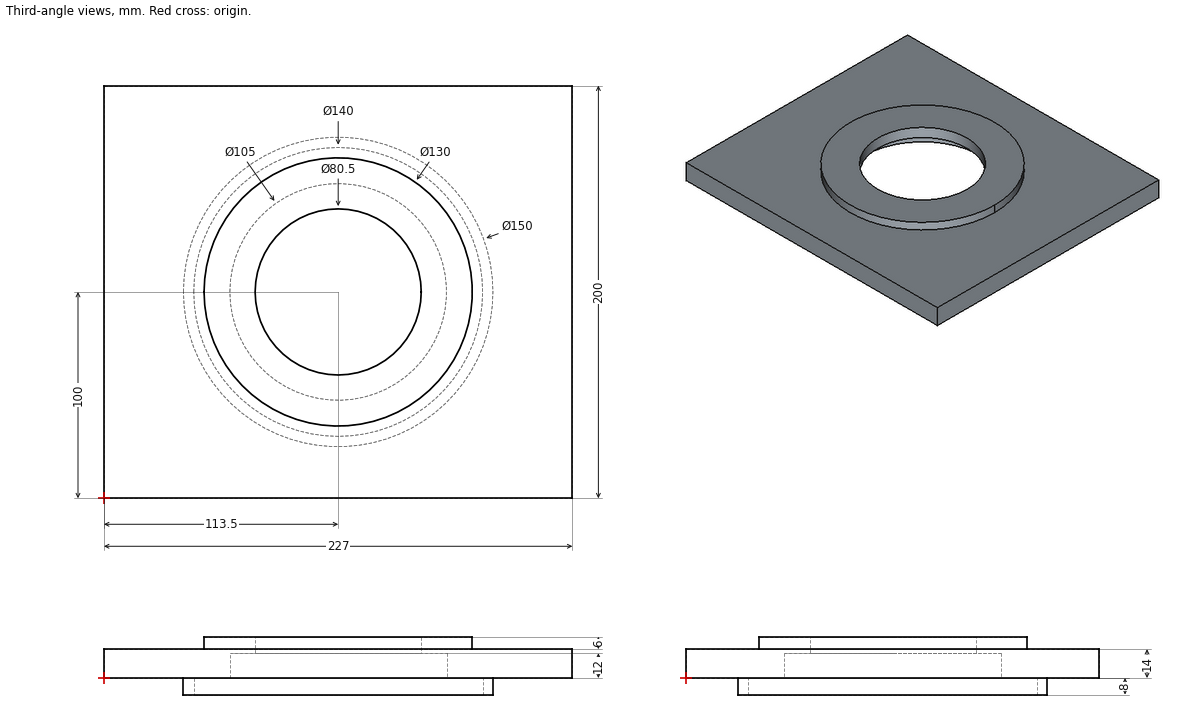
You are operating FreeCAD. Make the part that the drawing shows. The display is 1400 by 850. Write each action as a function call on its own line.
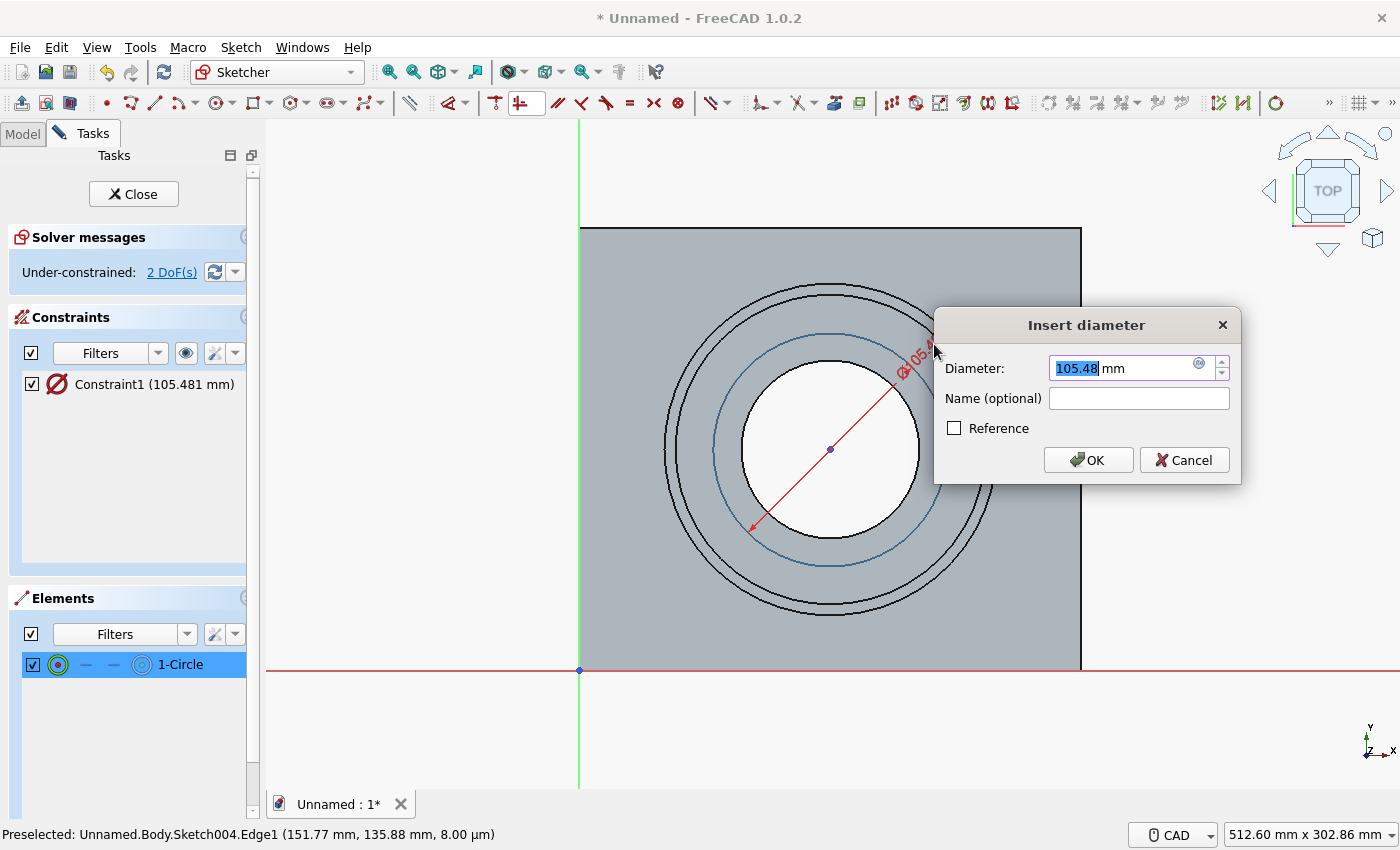
text(105)
key(Return)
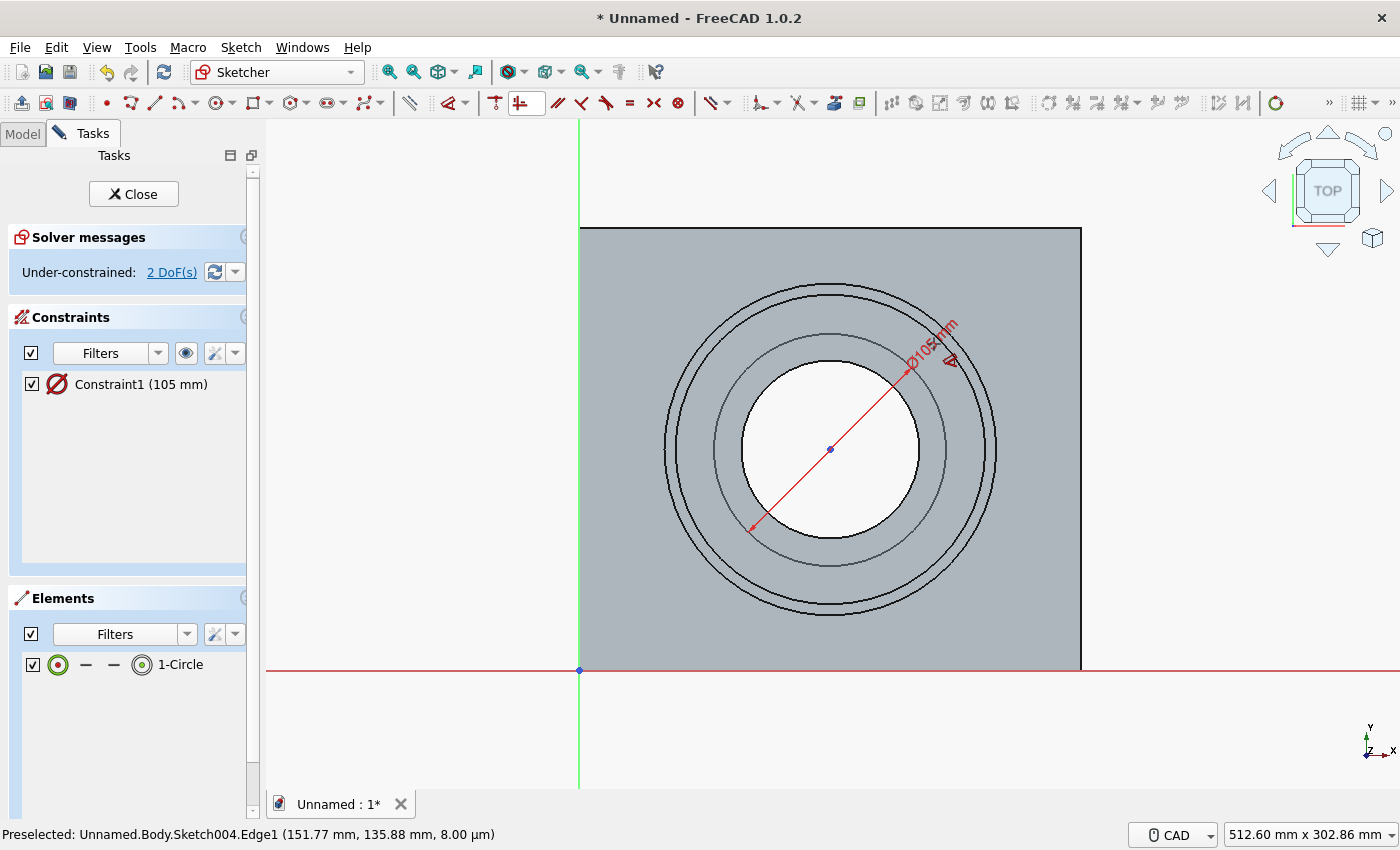
click(830, 450)
click(545, 560)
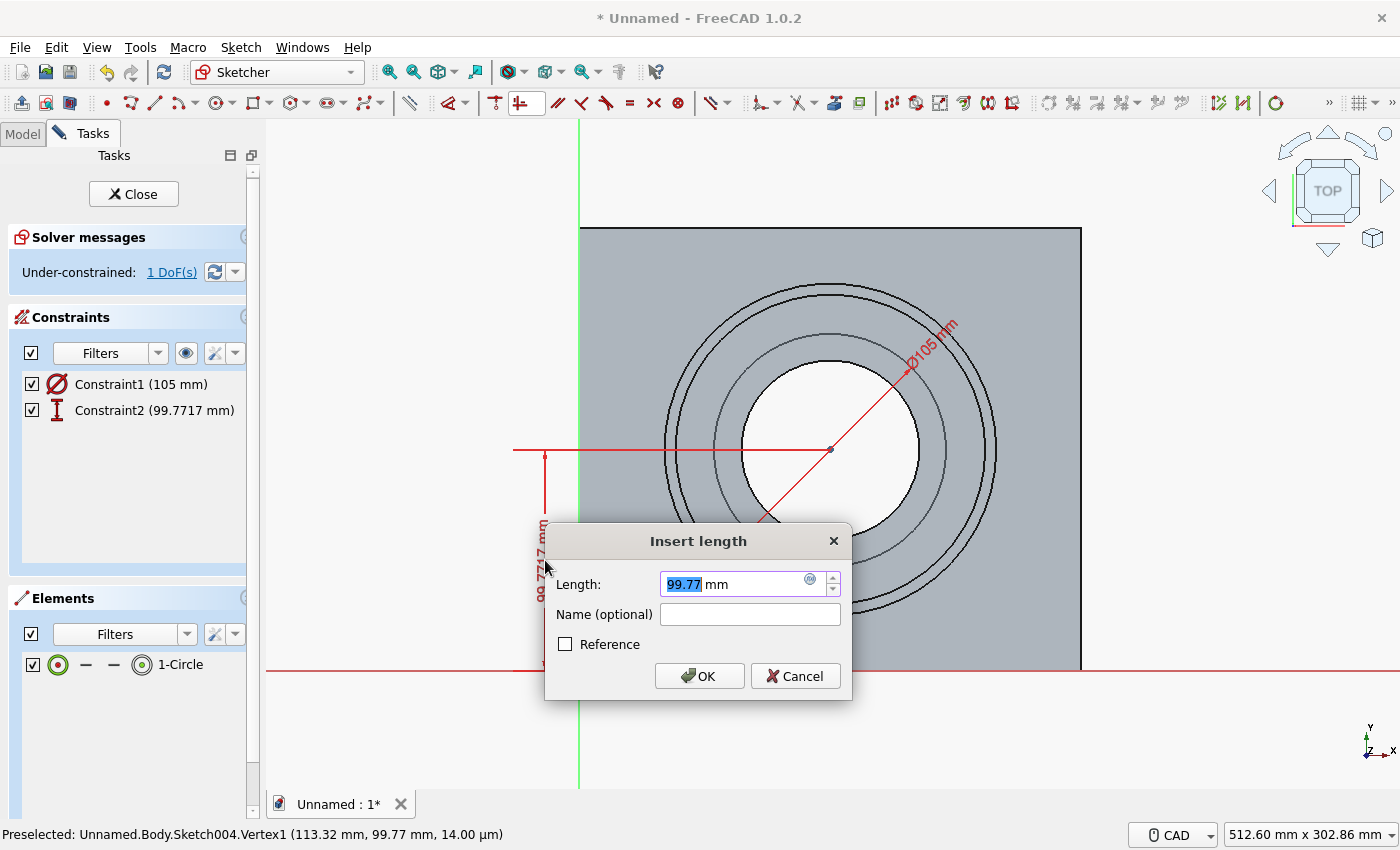
text(100)
key(Return)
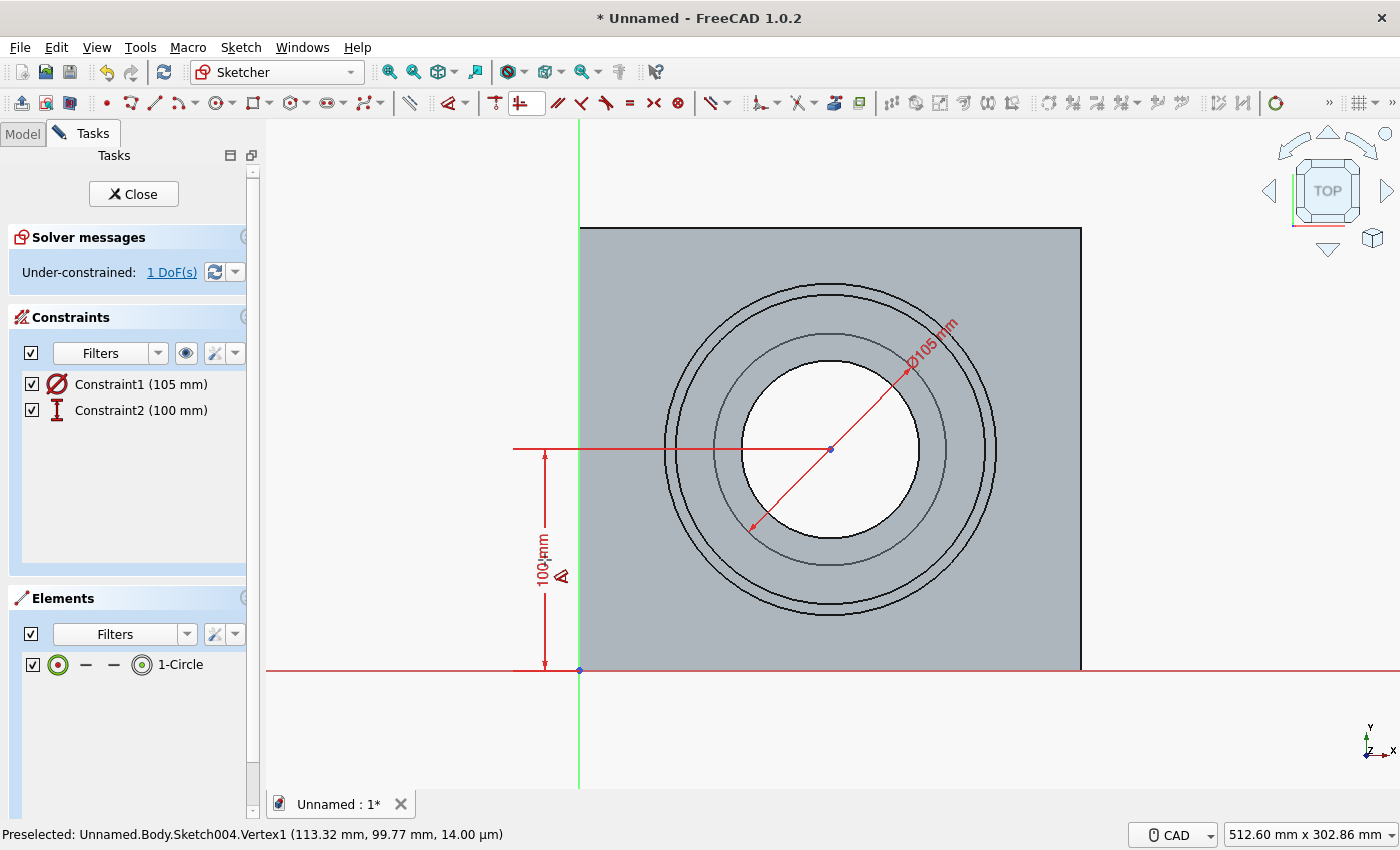
click(830, 449)
click(705, 705)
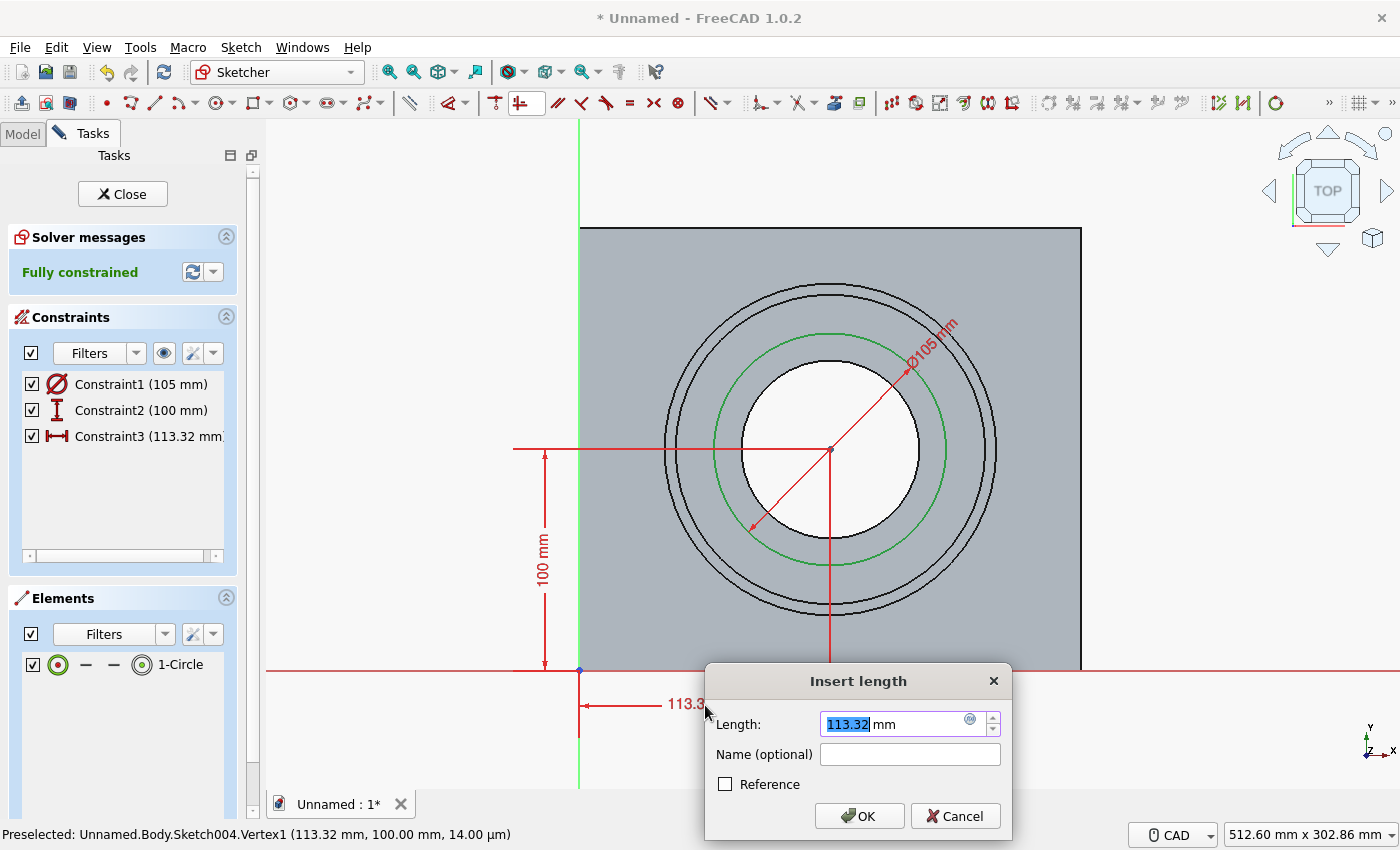
text(113.5)
key(Return)
key(Escape)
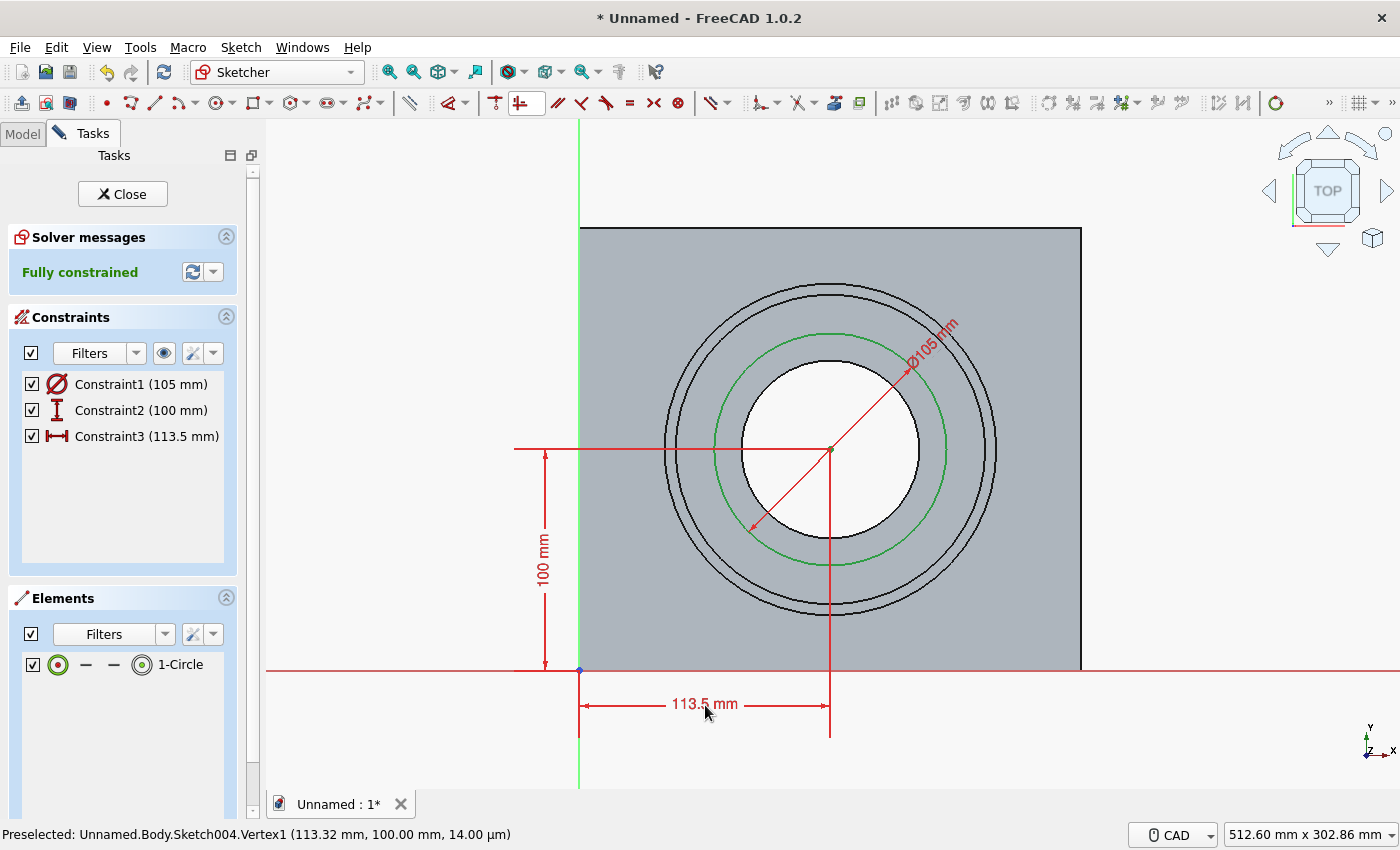
click(123, 194)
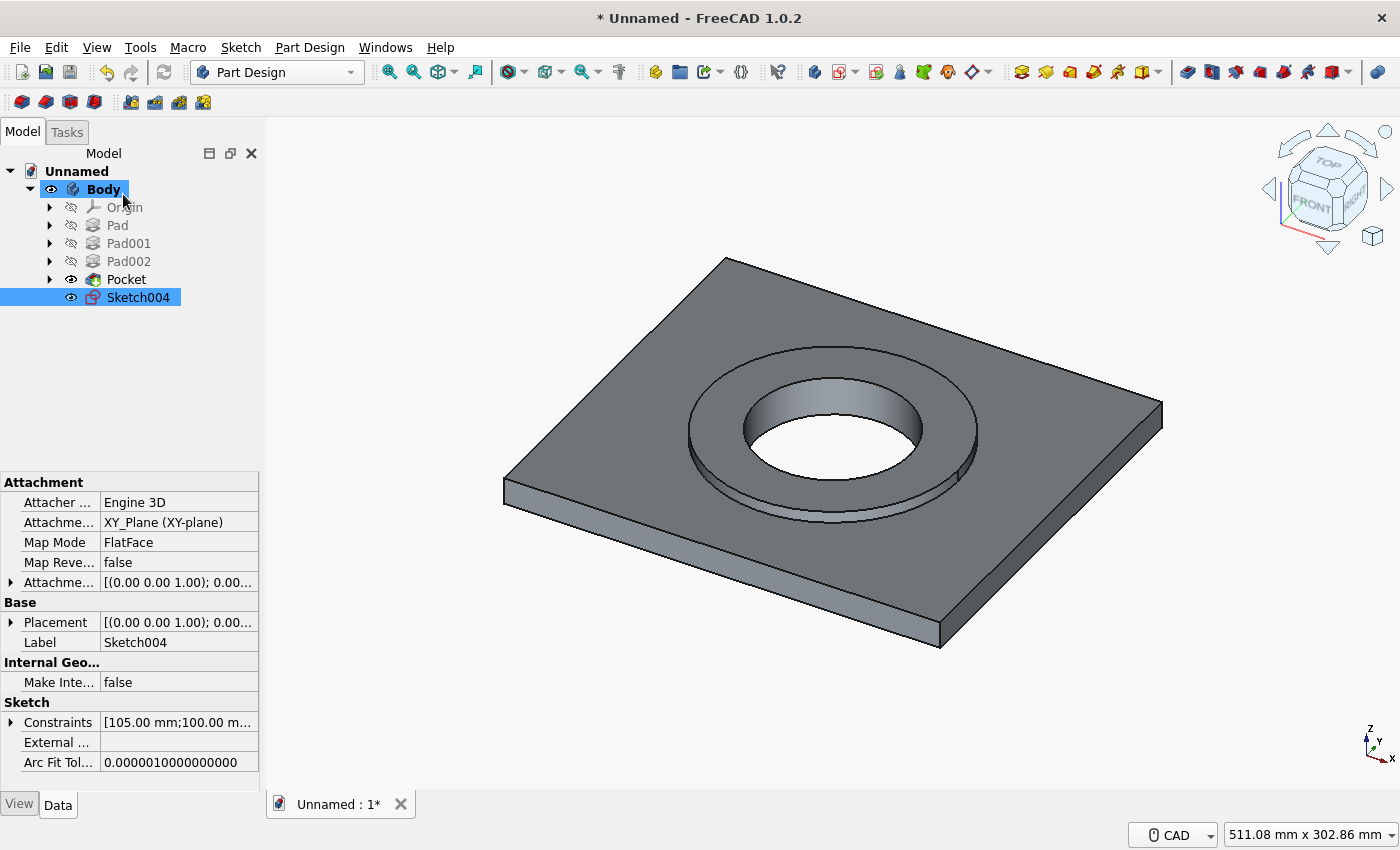
click(1188, 72)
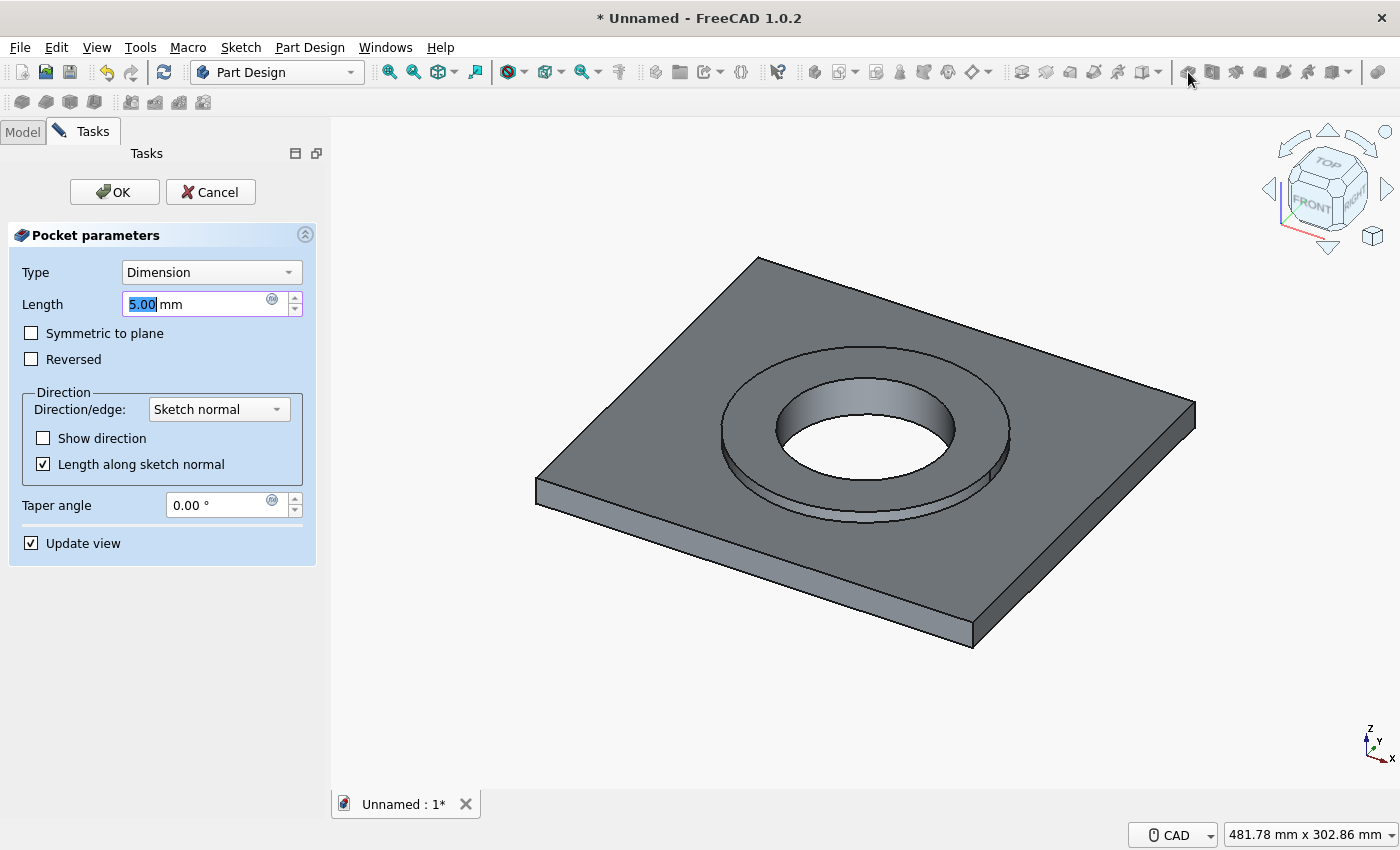
text(12)
key(Tab)